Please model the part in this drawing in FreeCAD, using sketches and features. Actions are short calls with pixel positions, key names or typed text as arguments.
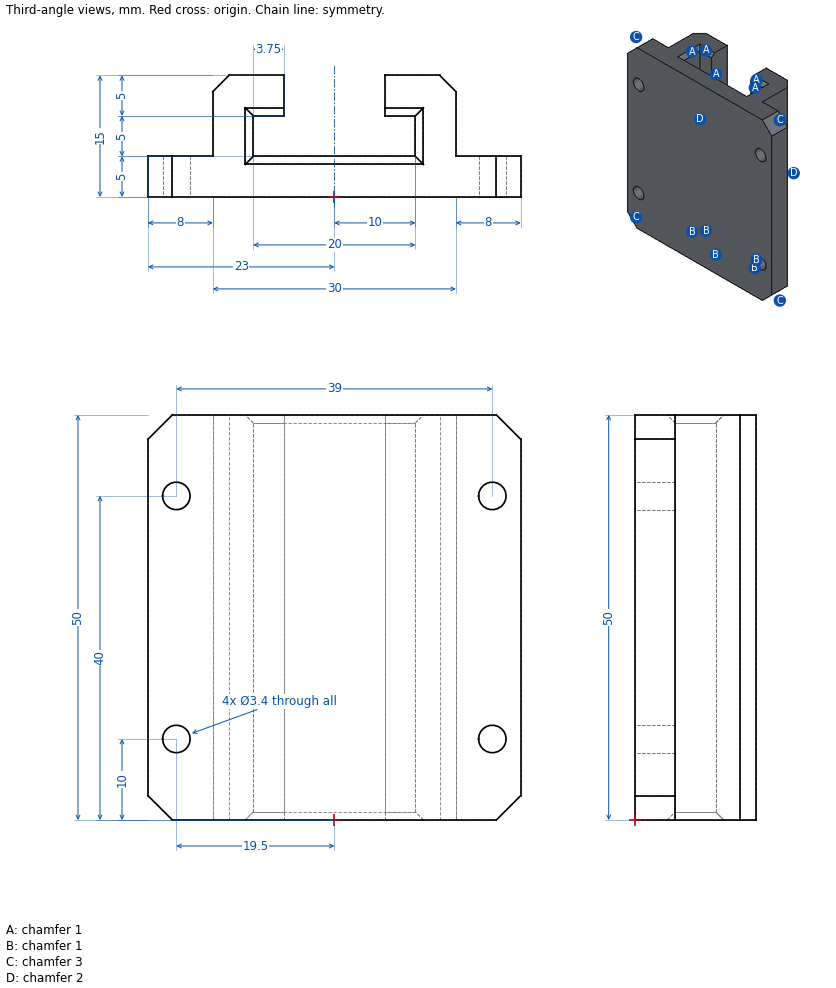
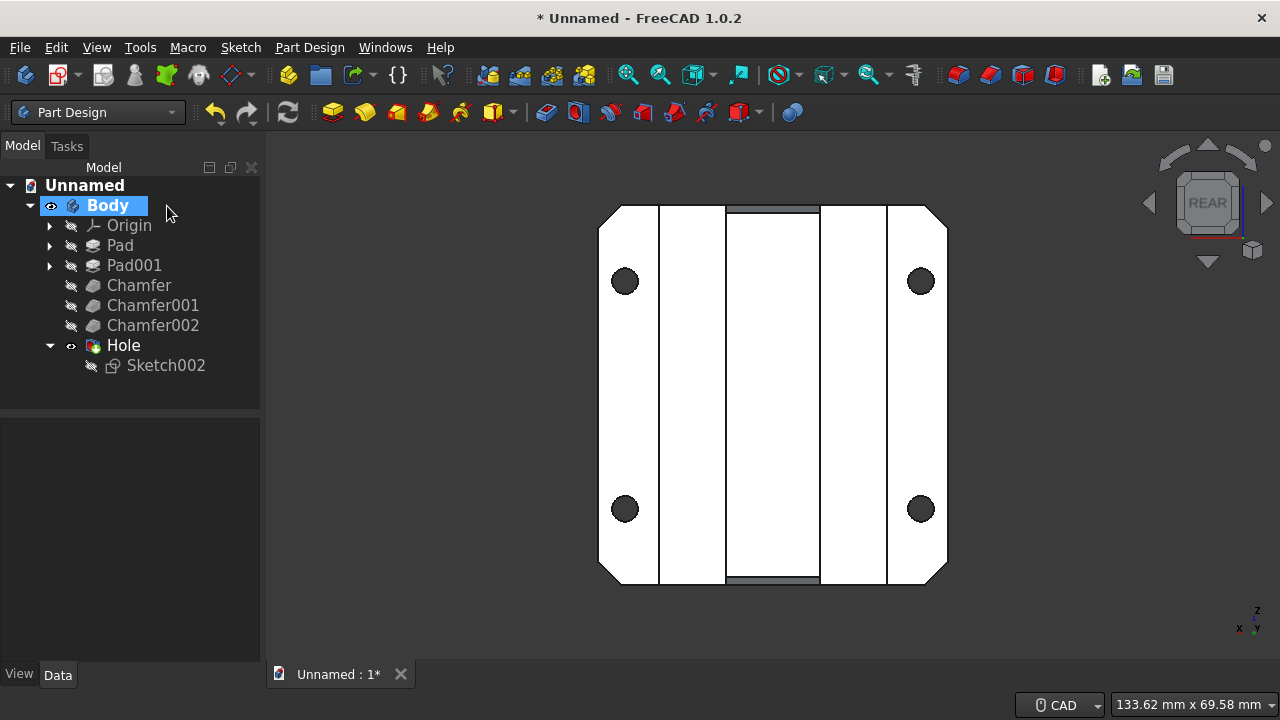
click(887, 394)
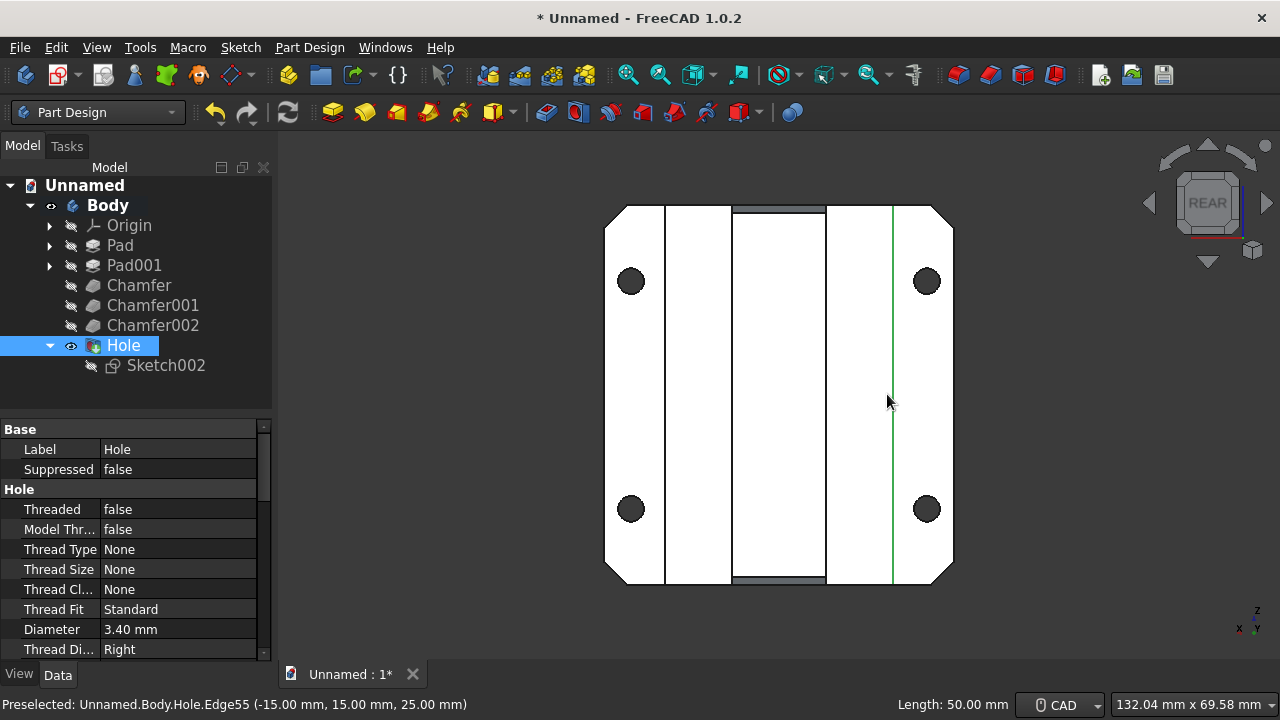
key(0)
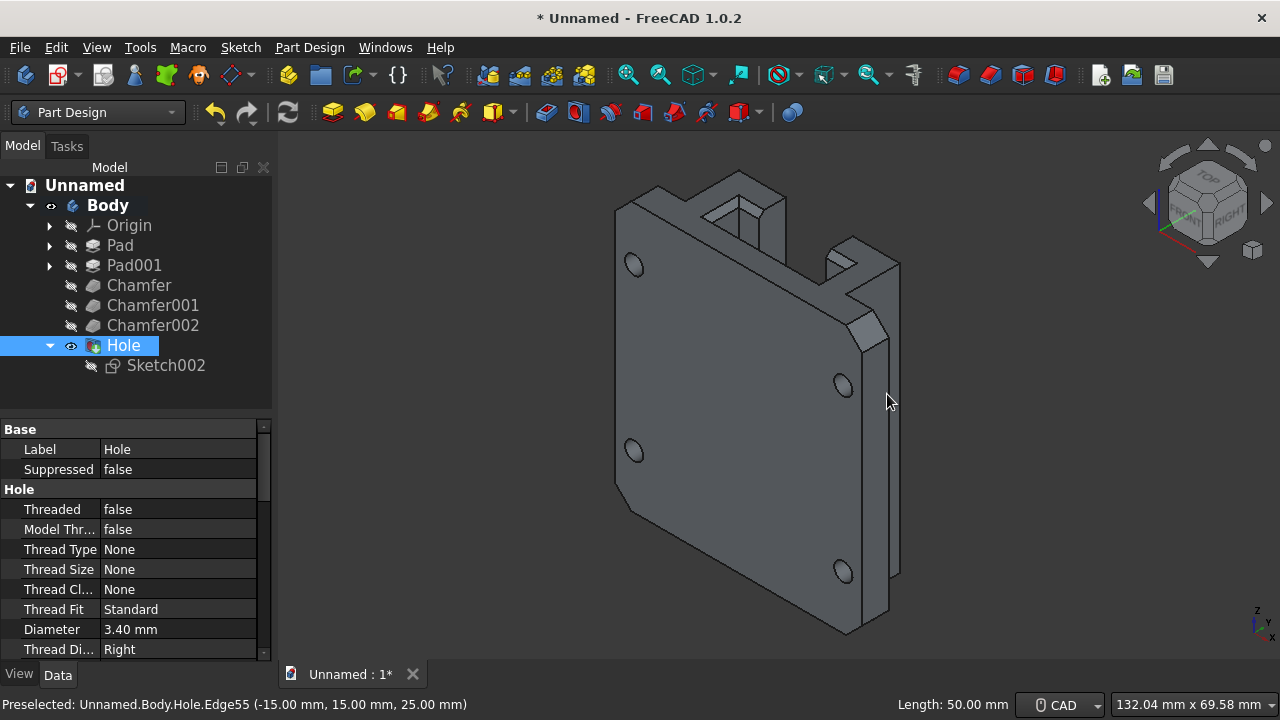
key(2)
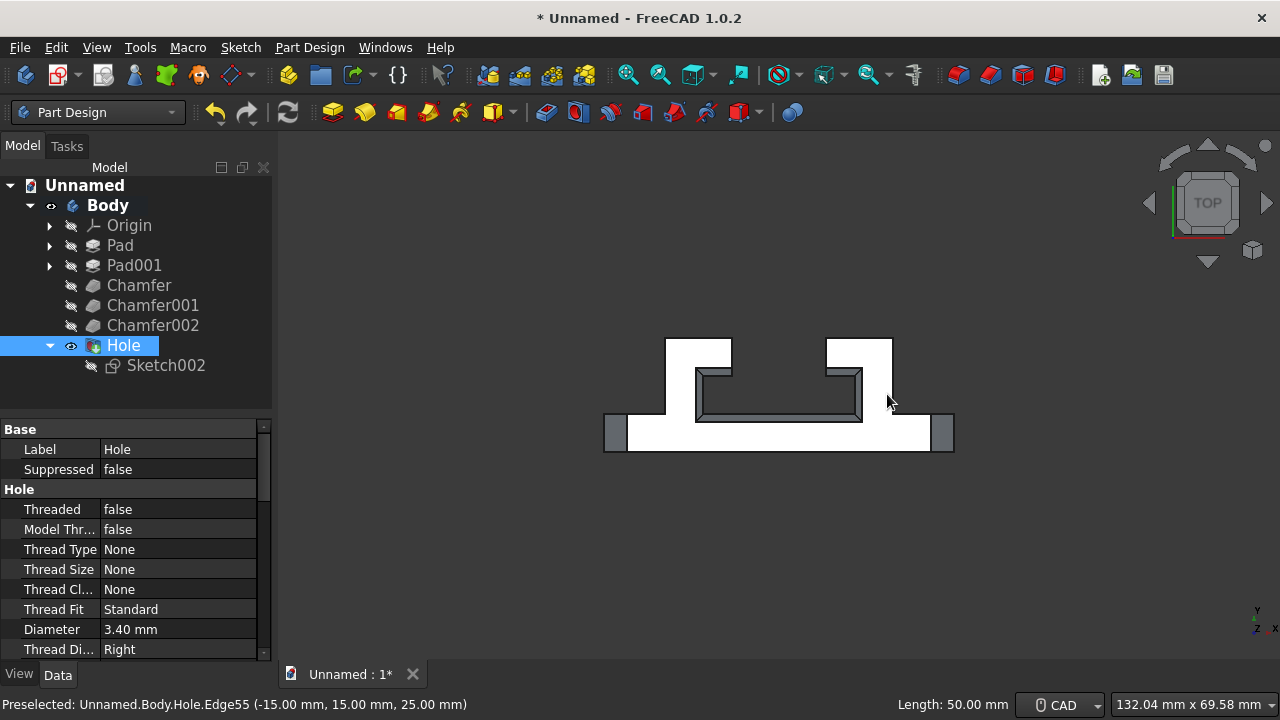
key(v)
key(f)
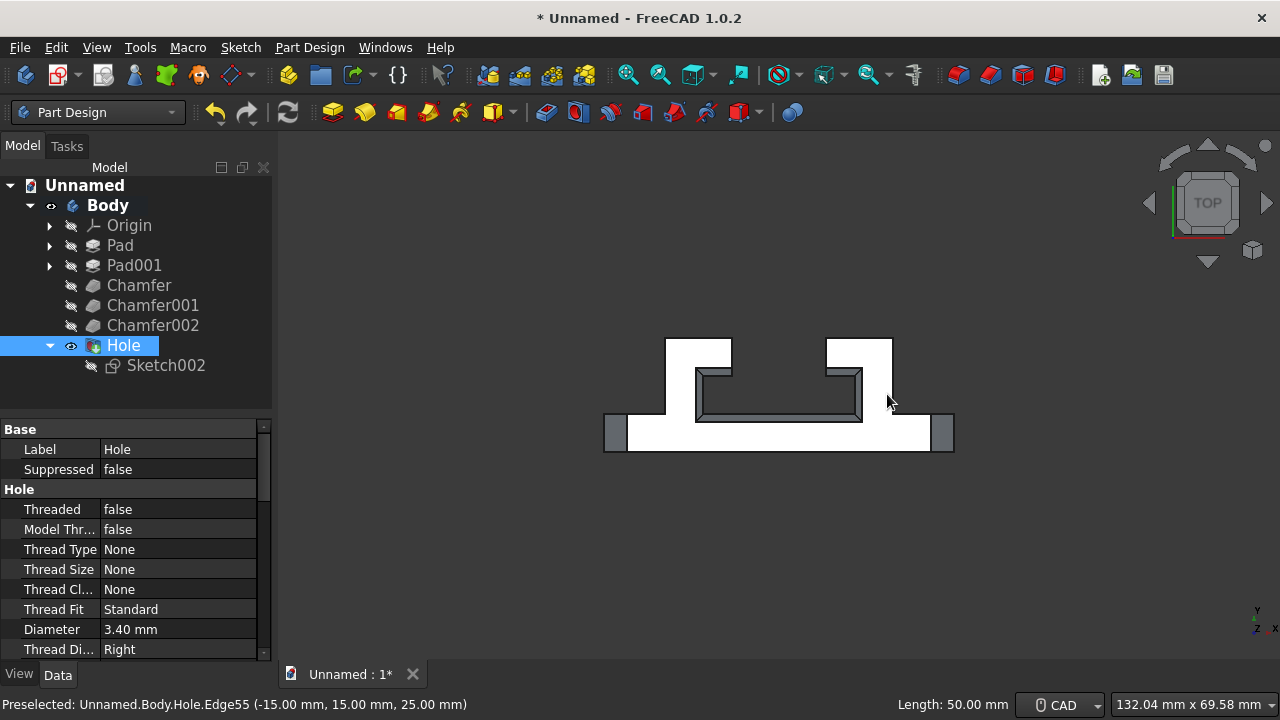
key(1)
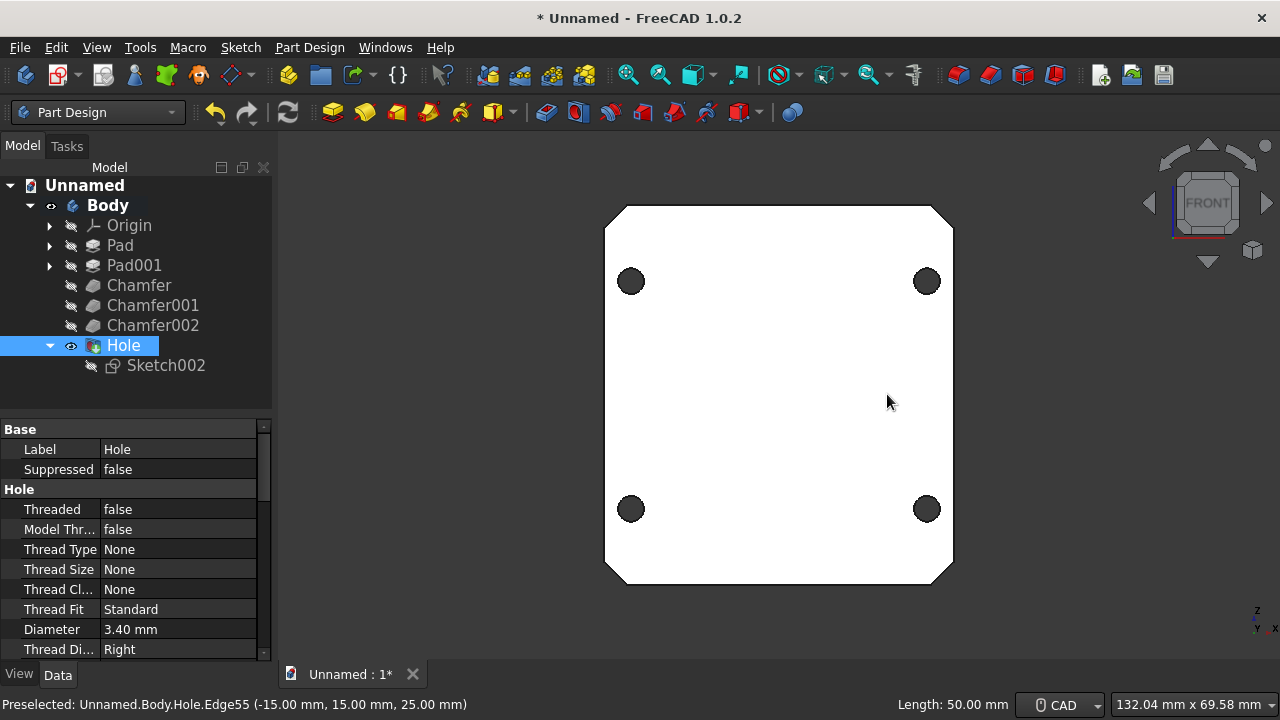
key(3)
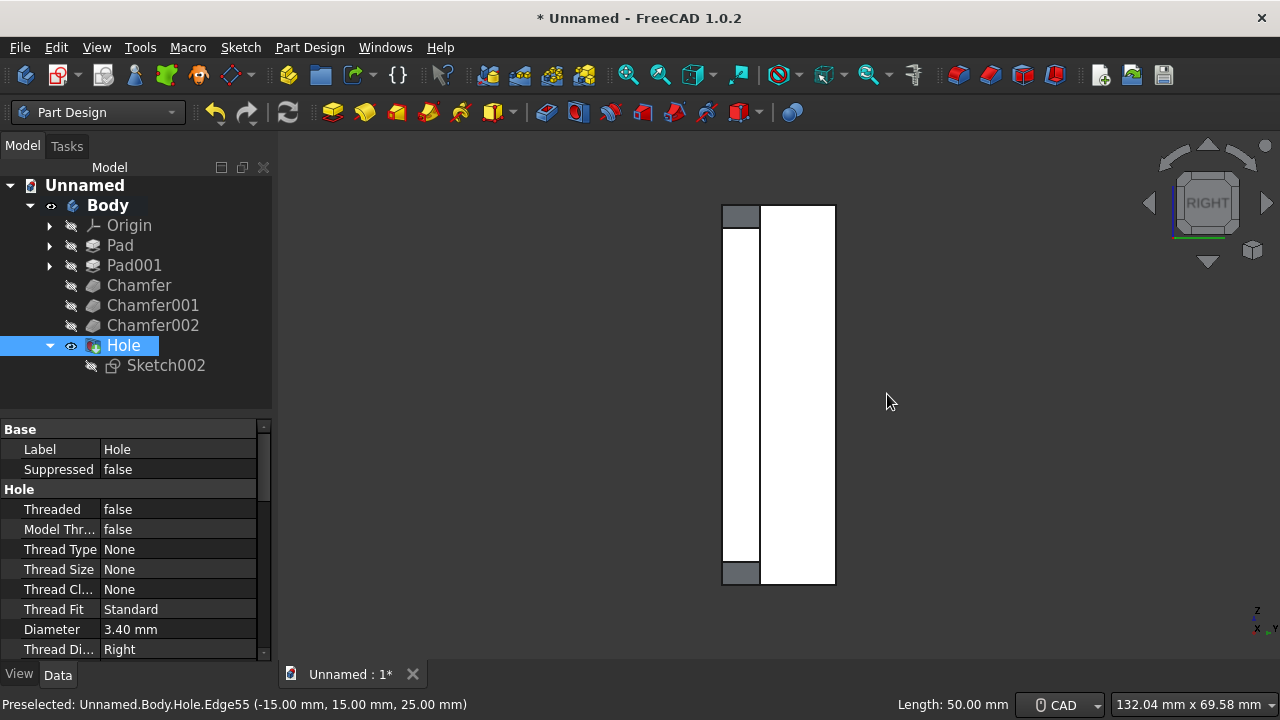
click(836, 394, ctrl)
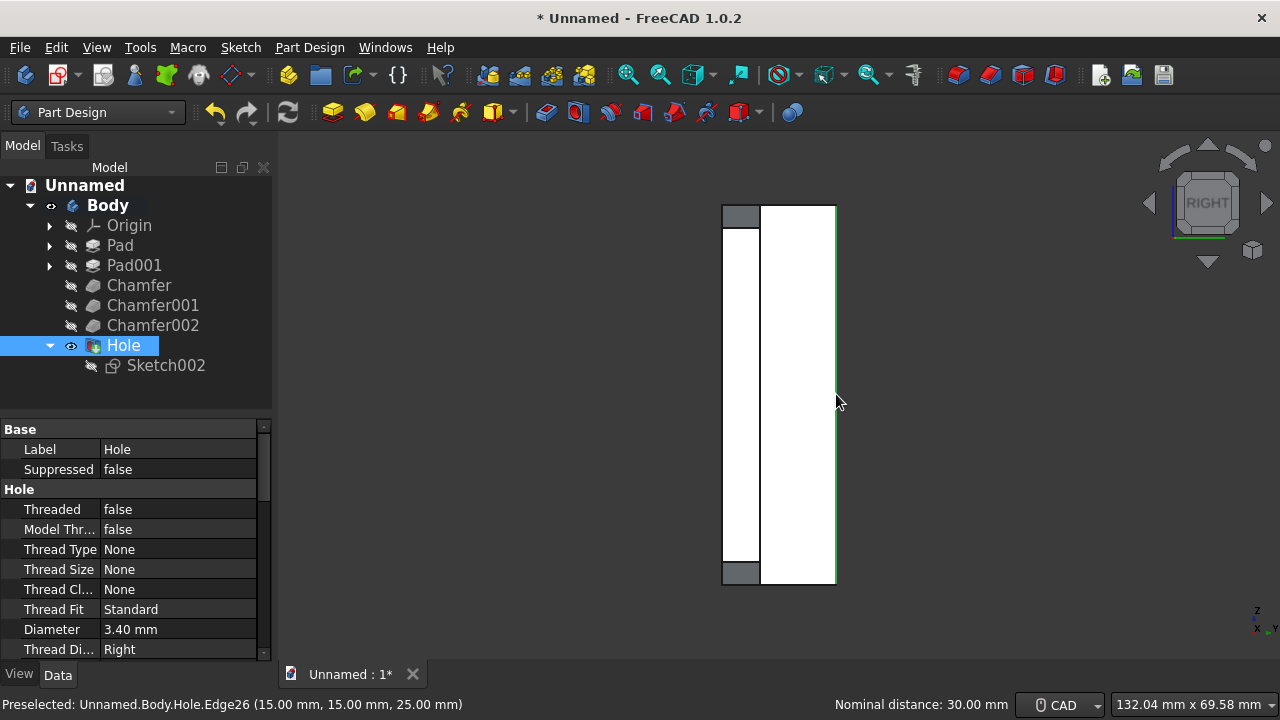
click(992, 76)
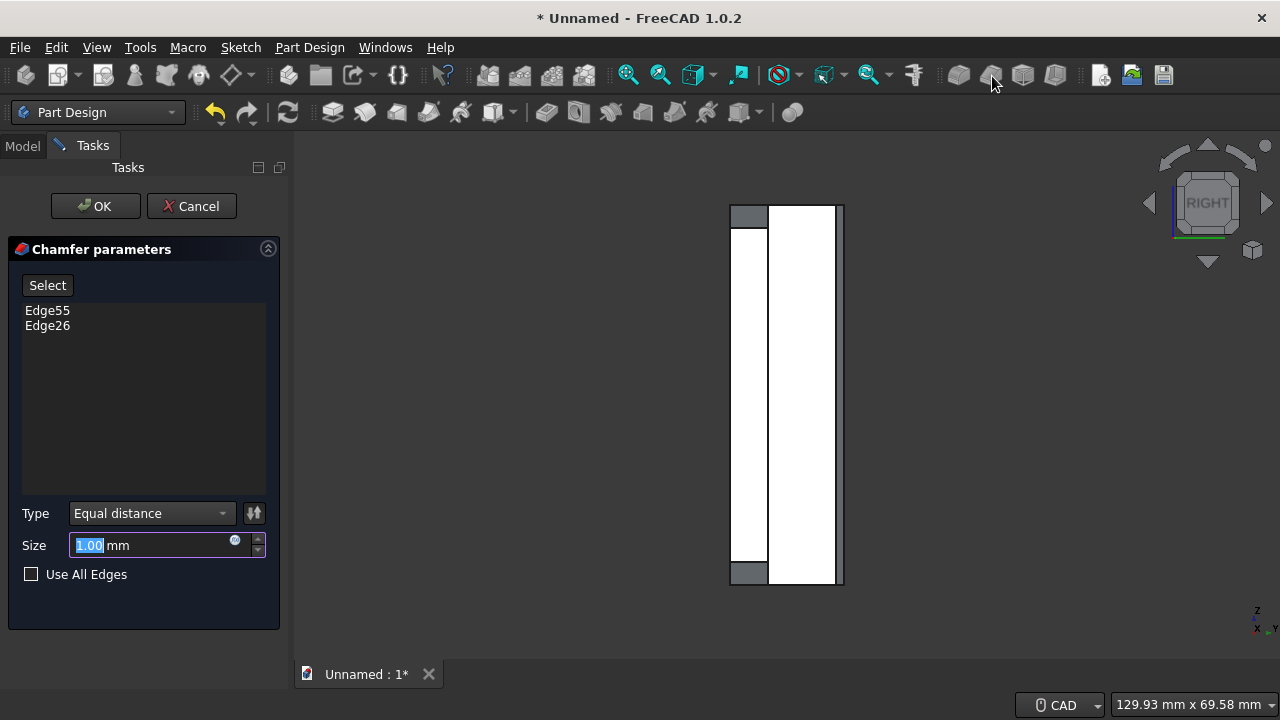
text(2)
key(Tab)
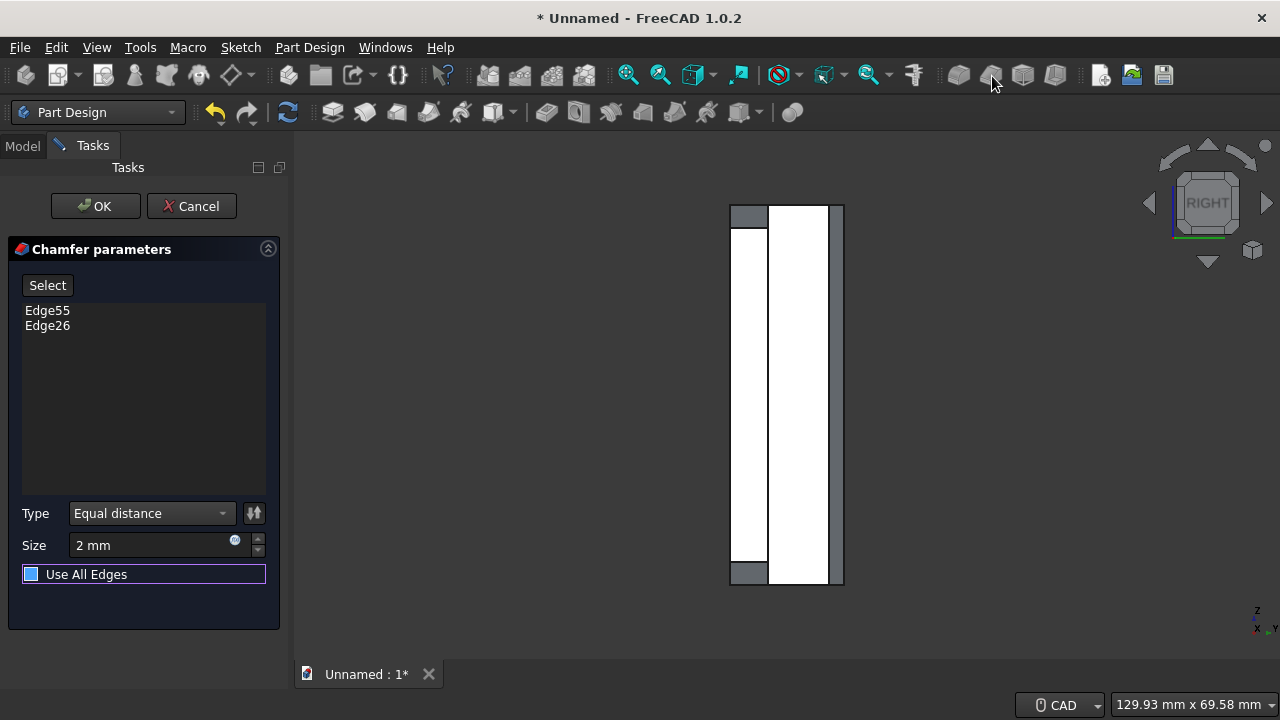
click(96, 206)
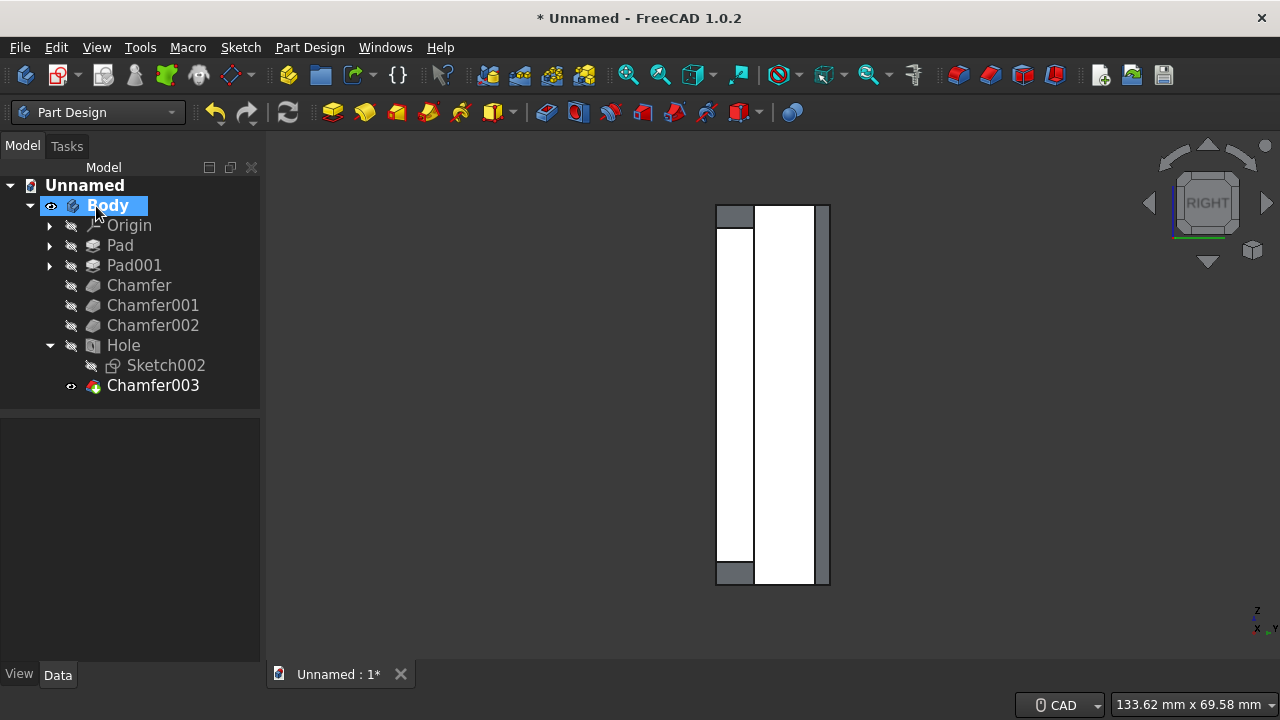
key(0)